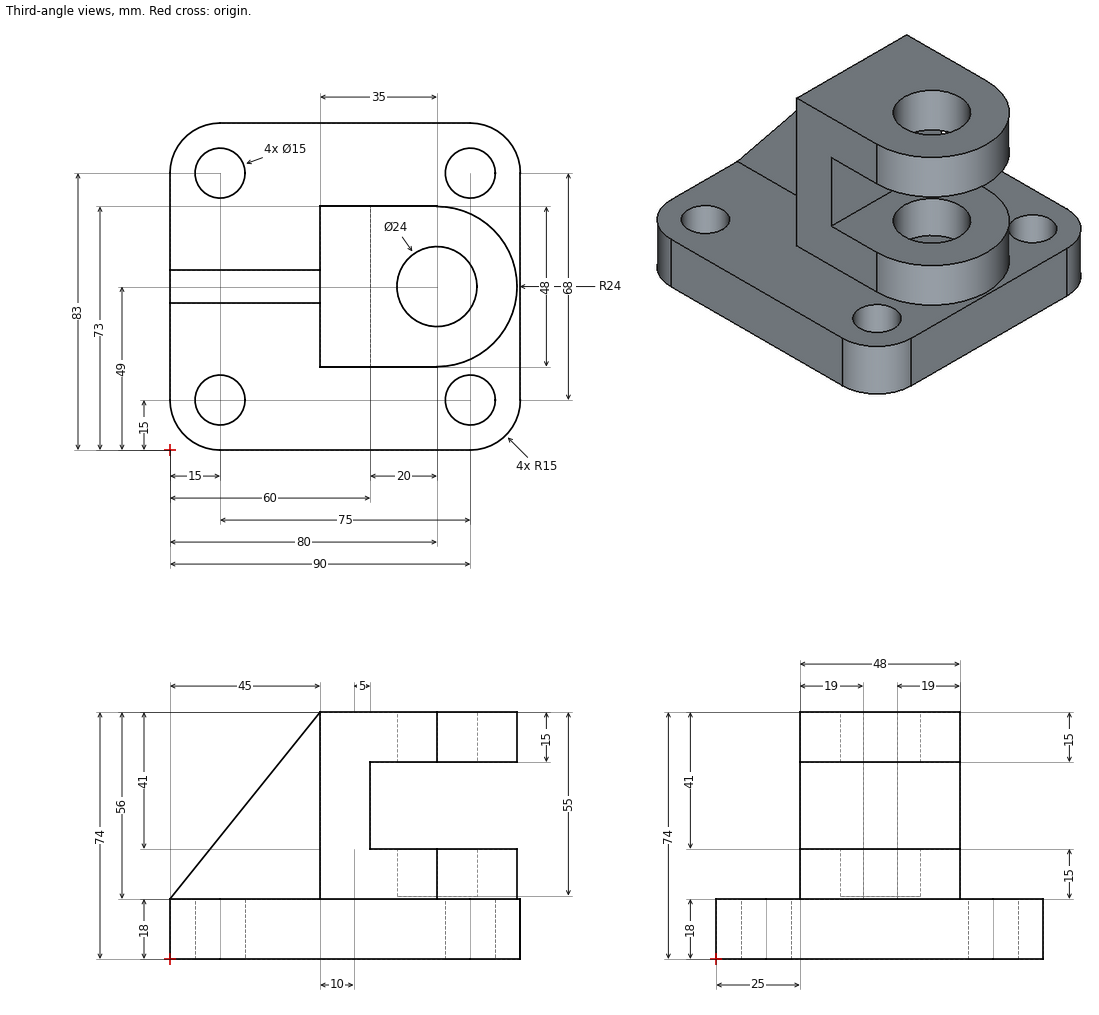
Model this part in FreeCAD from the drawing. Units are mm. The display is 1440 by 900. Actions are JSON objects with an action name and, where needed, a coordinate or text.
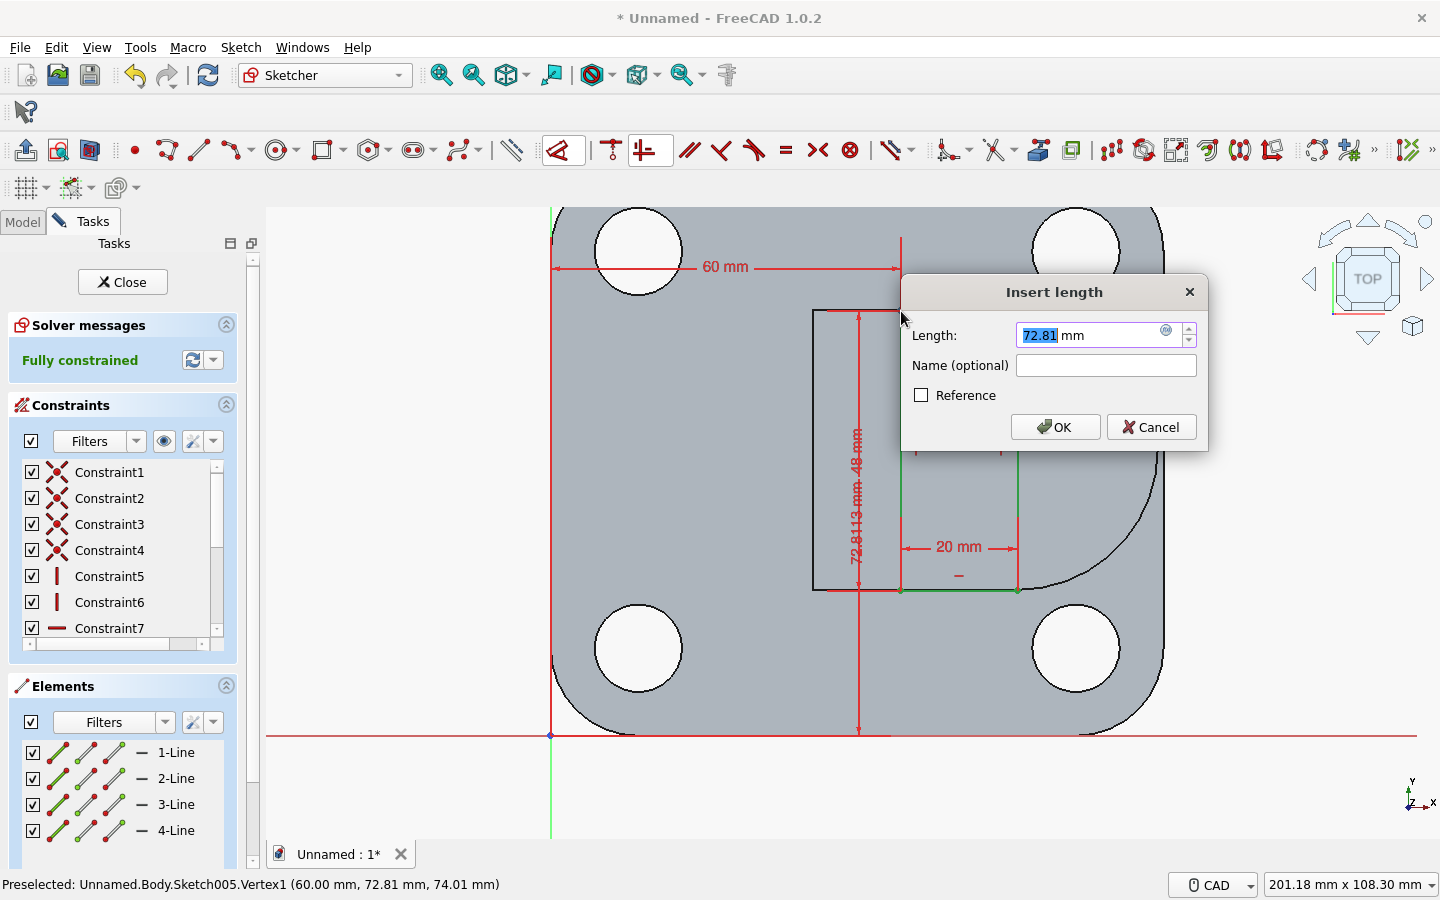
{"action": "type", "text": "73"}
{"action": "key", "text": "Return"}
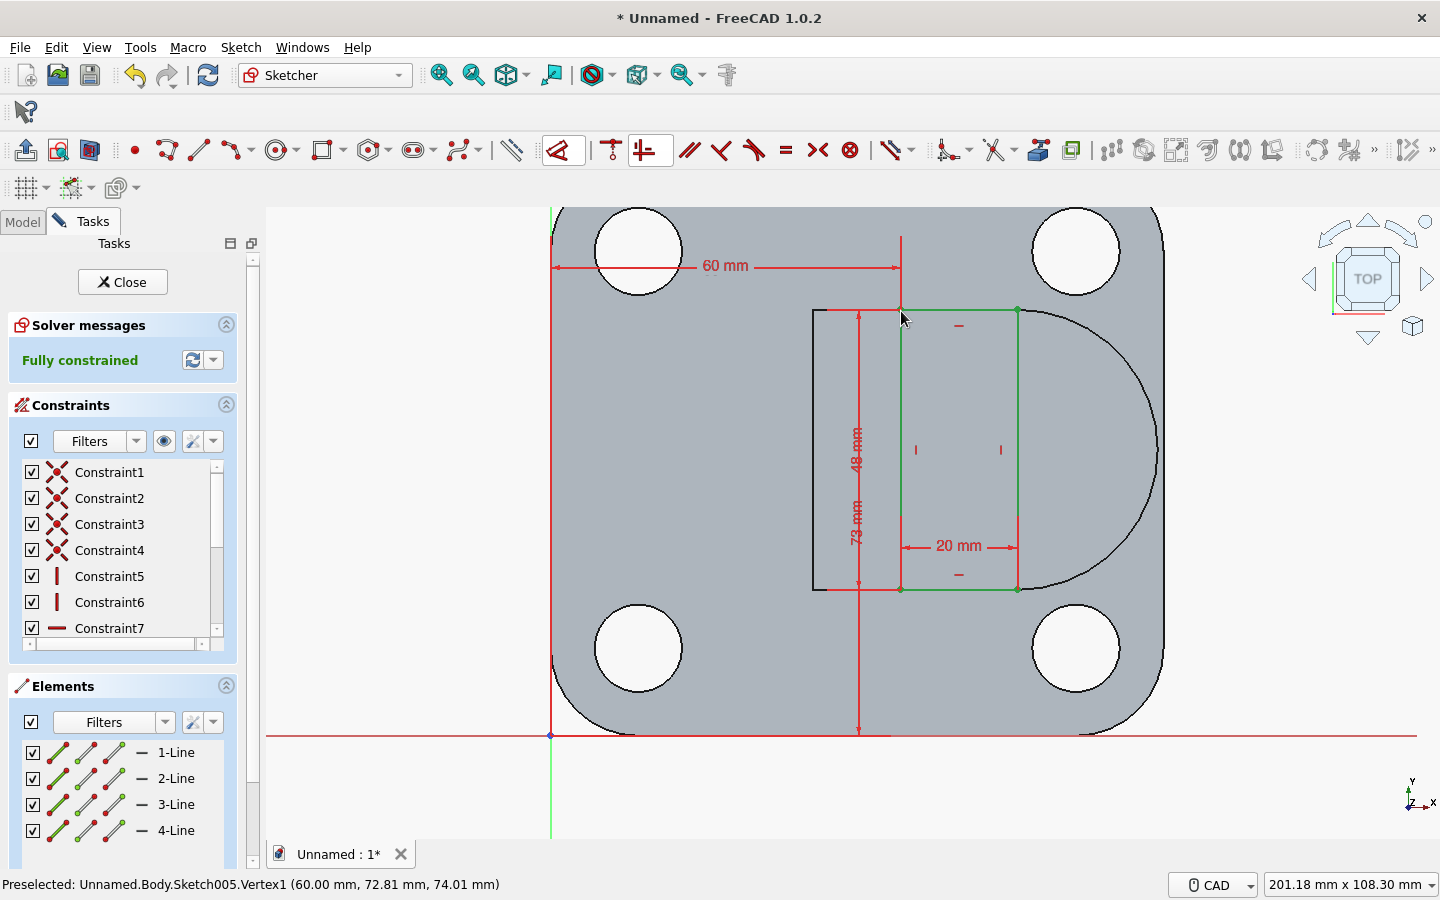
{"action": "left_click", "coordinate": [123, 282]}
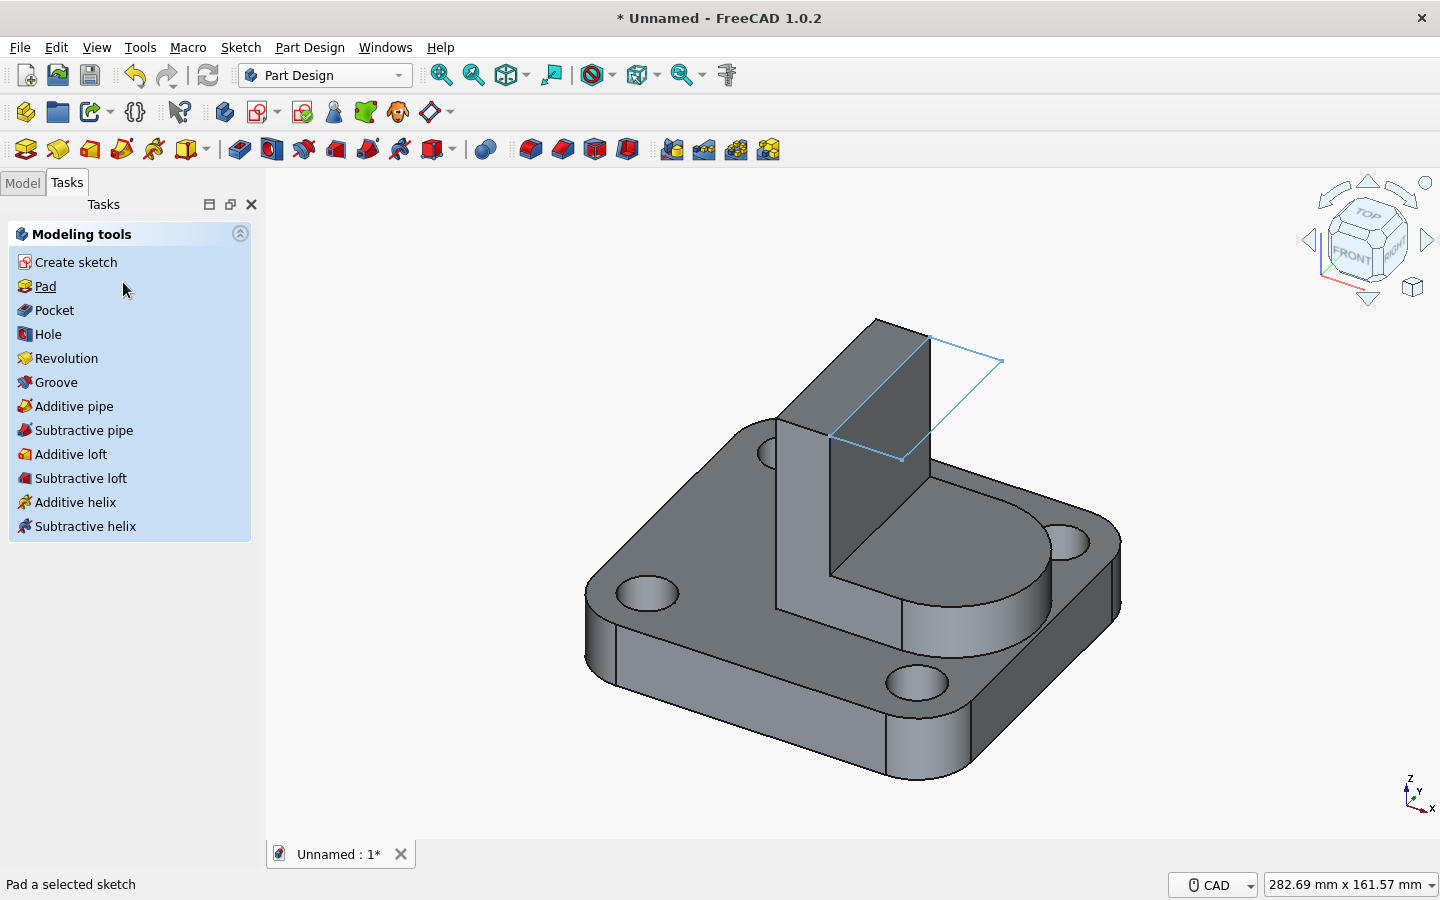
{"action": "left_click", "coordinate": [26, 150]}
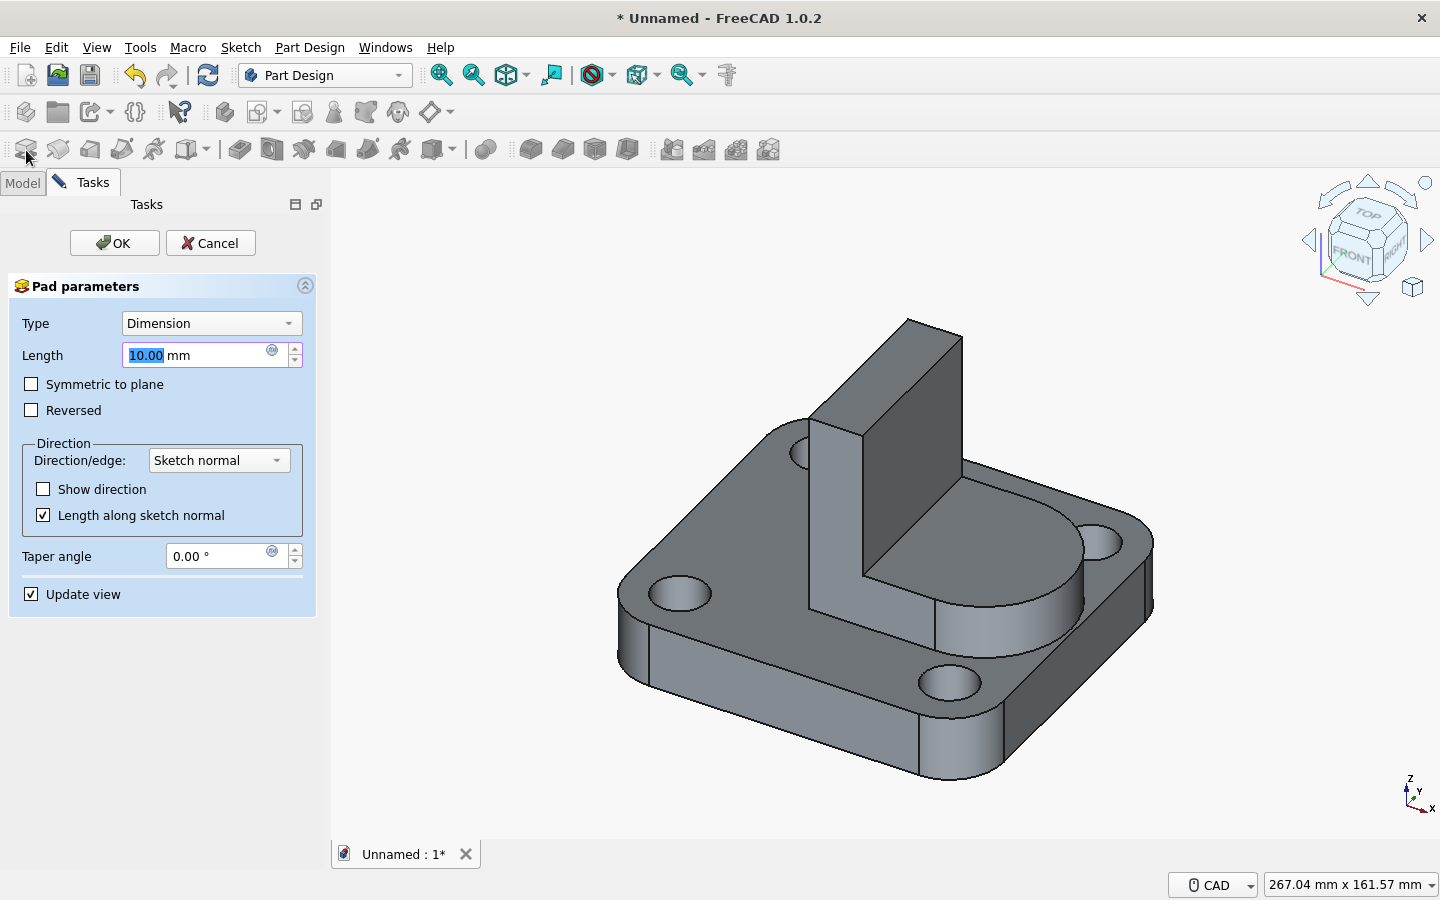
{"action": "type", "text": "15"}
{"action": "key", "text": "Tab"}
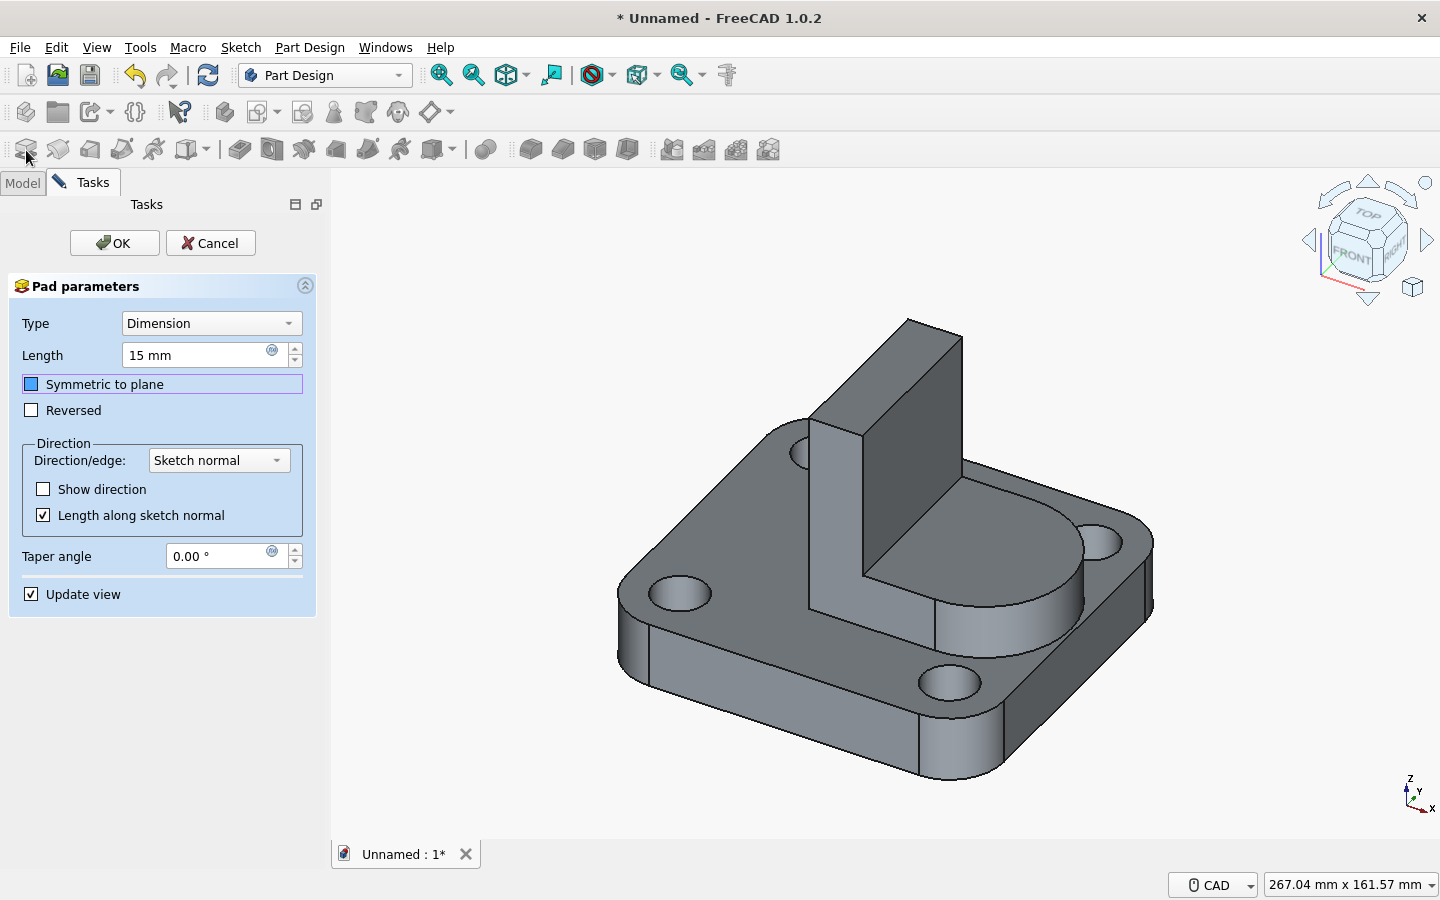
{"action": "left_click", "coordinate": [30, 410]}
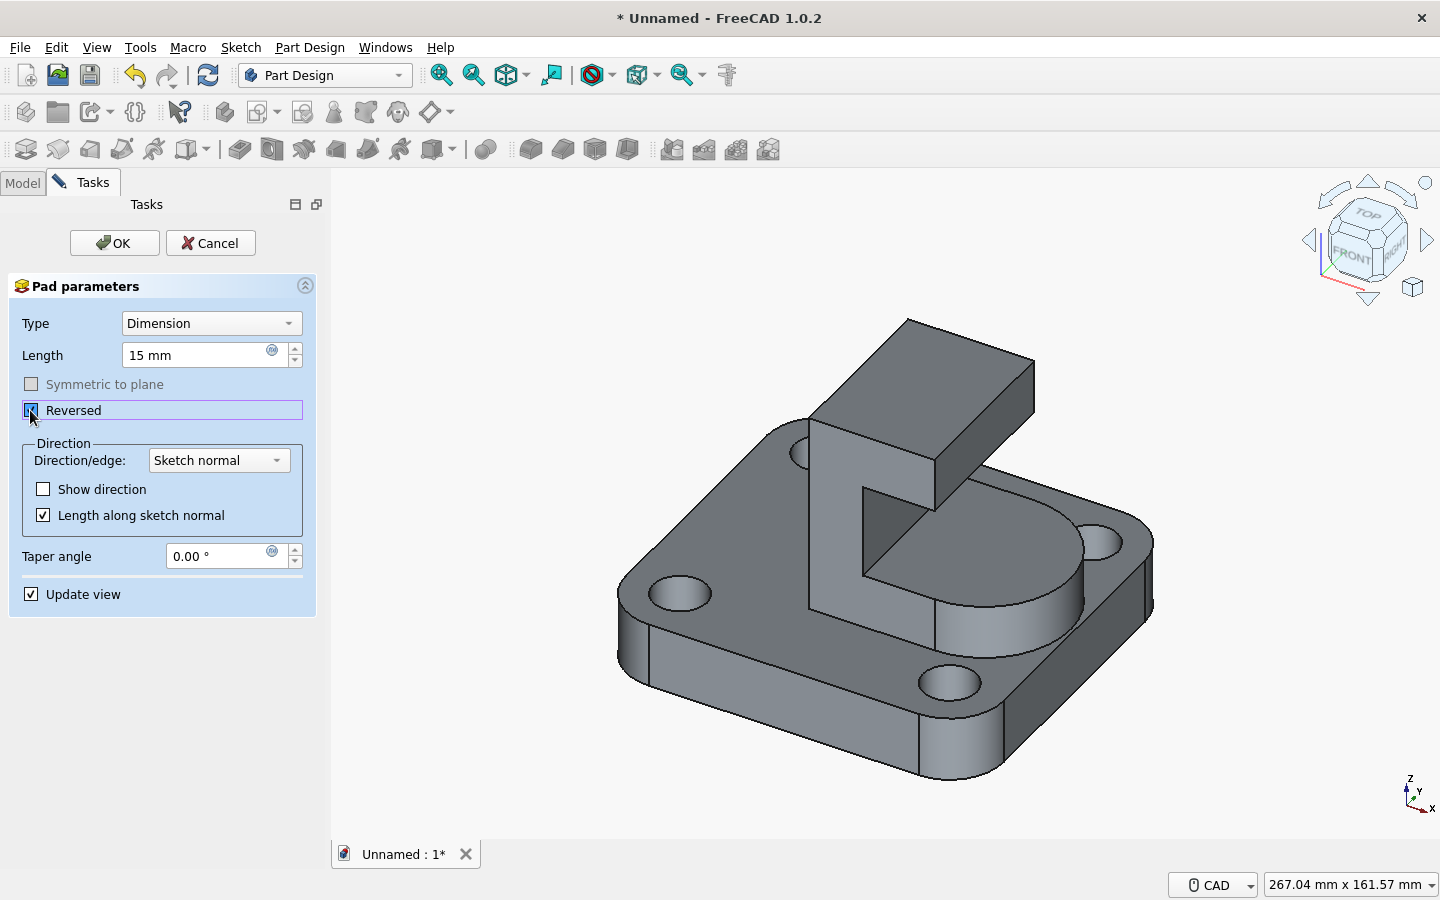
{"action": "left_click", "coordinate": [115, 243]}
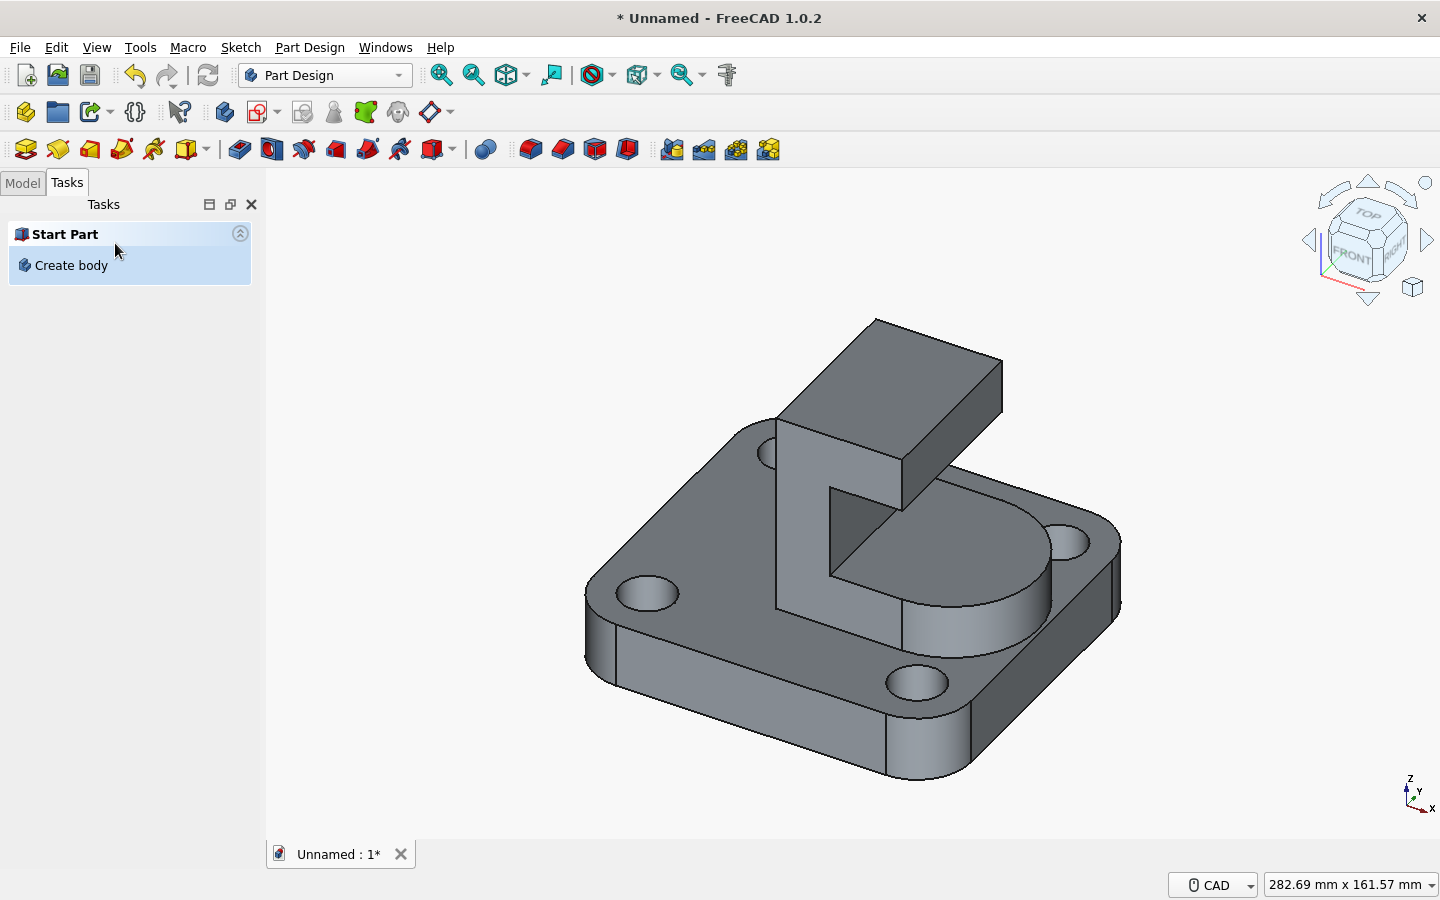
{"action": "left_click", "coordinate": [23, 182]}